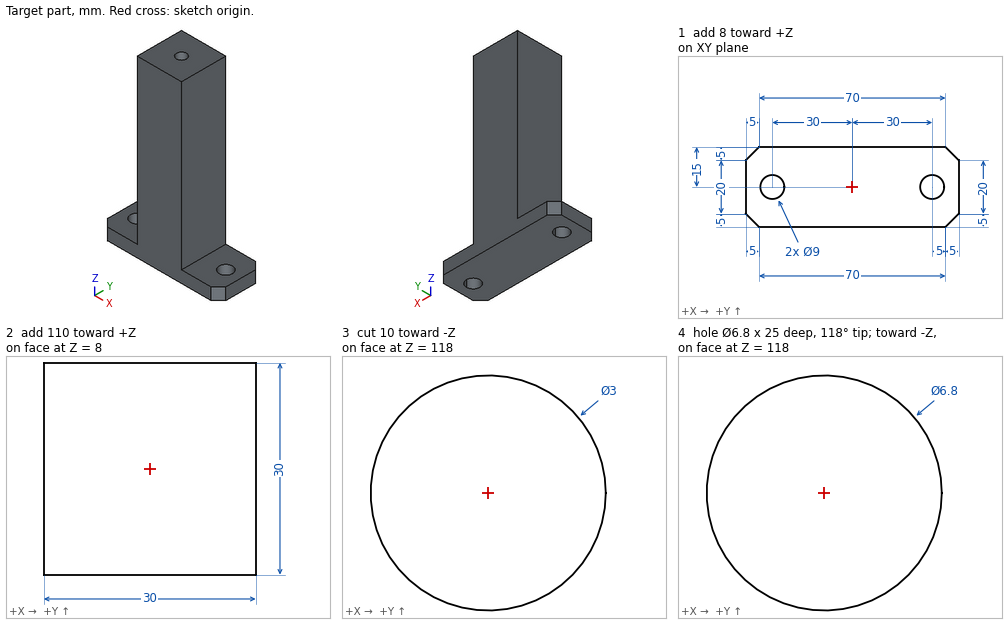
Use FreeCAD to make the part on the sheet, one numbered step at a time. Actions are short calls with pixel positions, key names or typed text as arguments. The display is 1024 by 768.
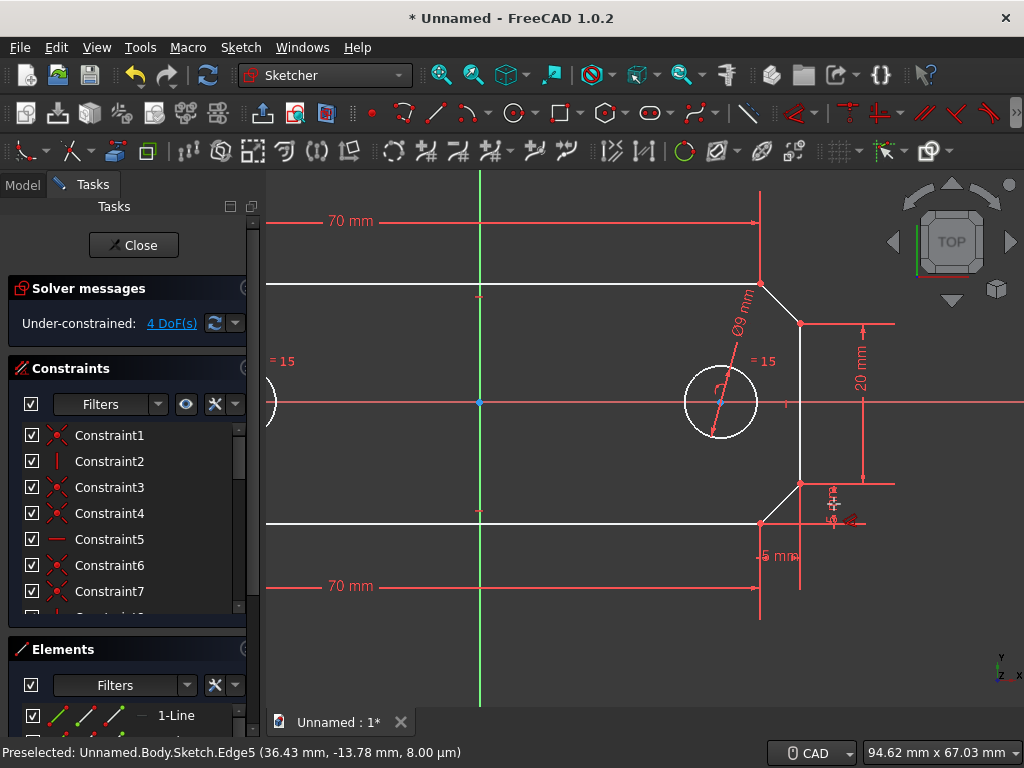
click(721, 402)
click(600, 436)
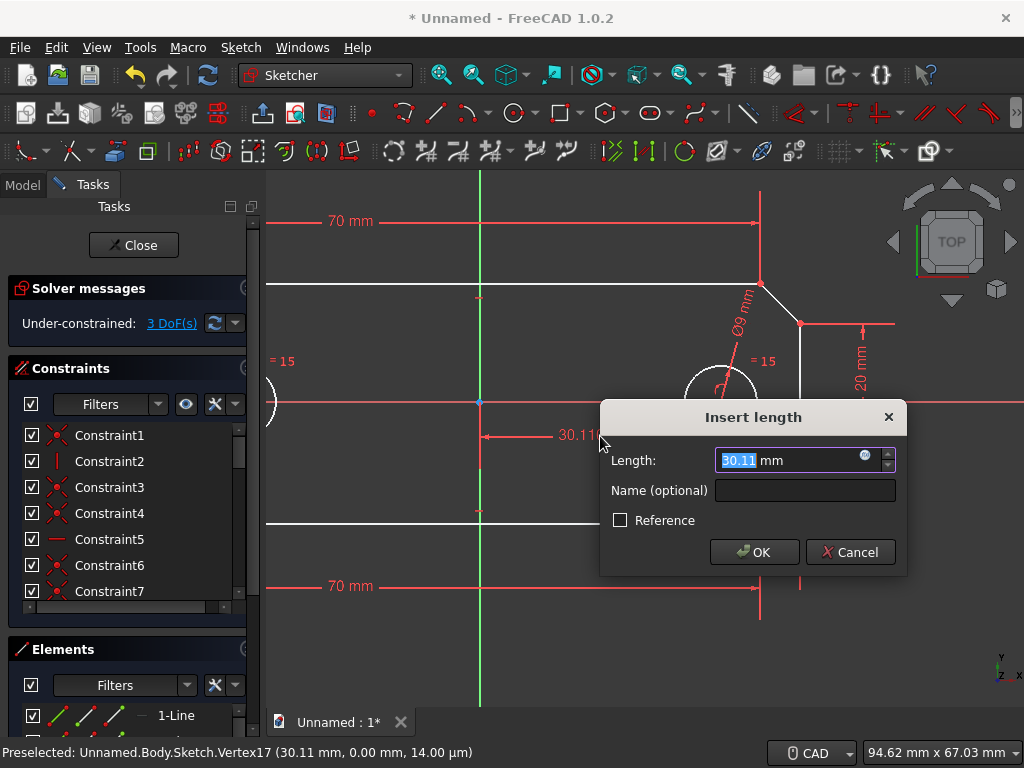
text(30)
key(Return)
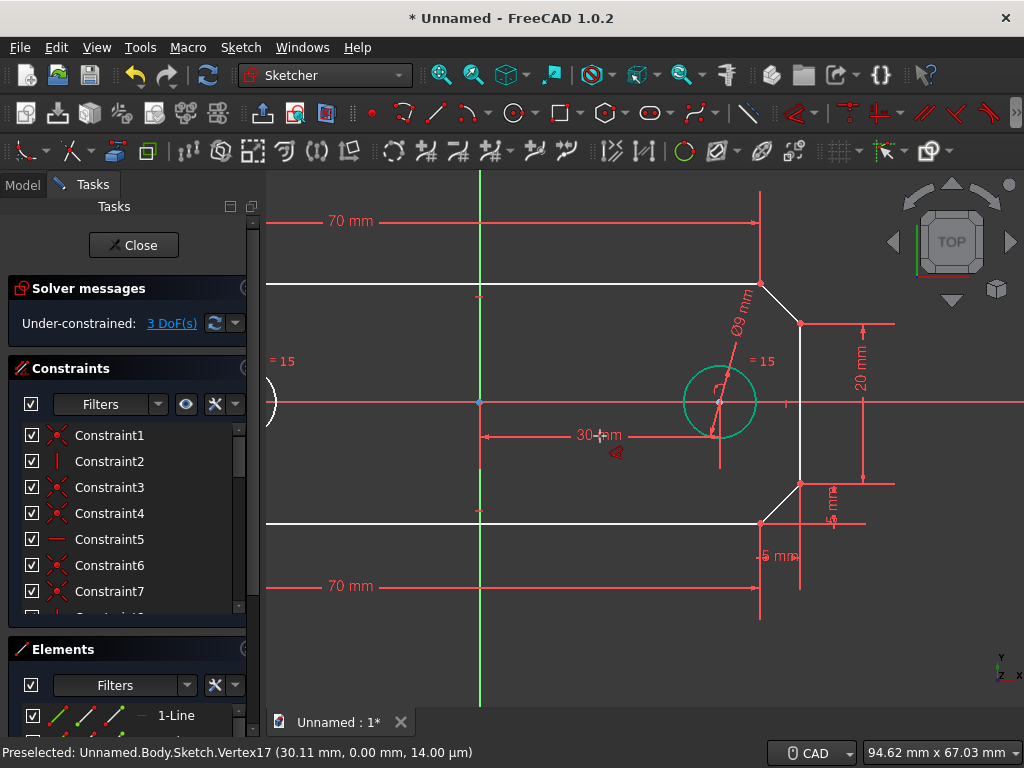
scroll(774, 513, down, 2)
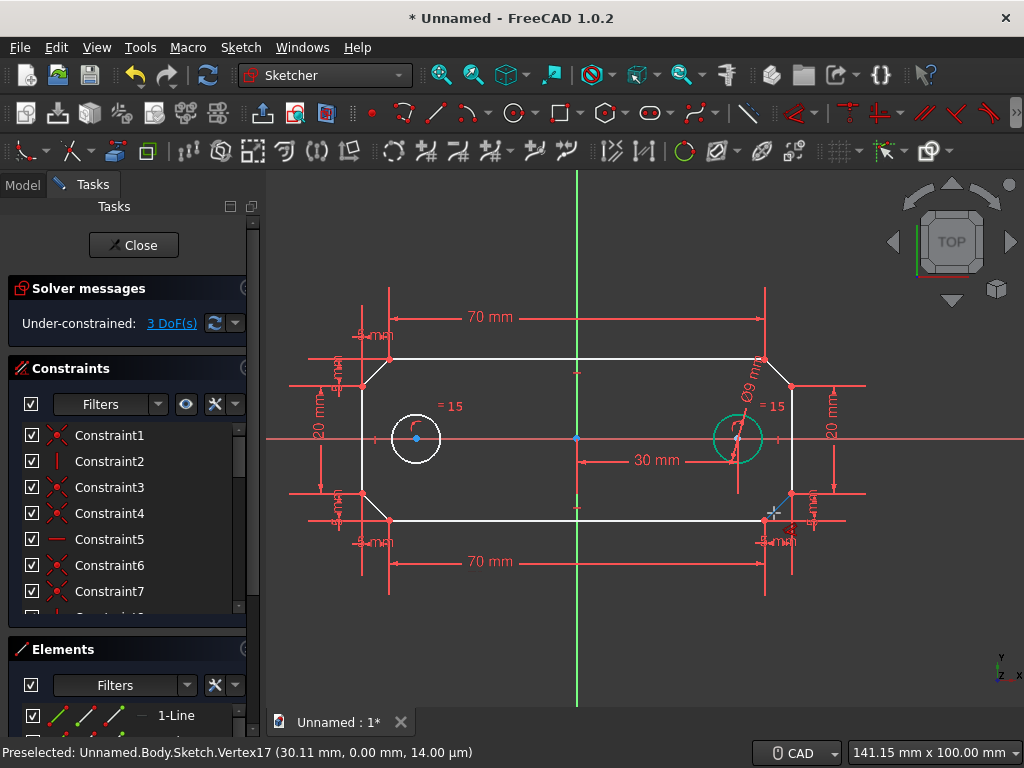
click(416, 439)
click(496, 473)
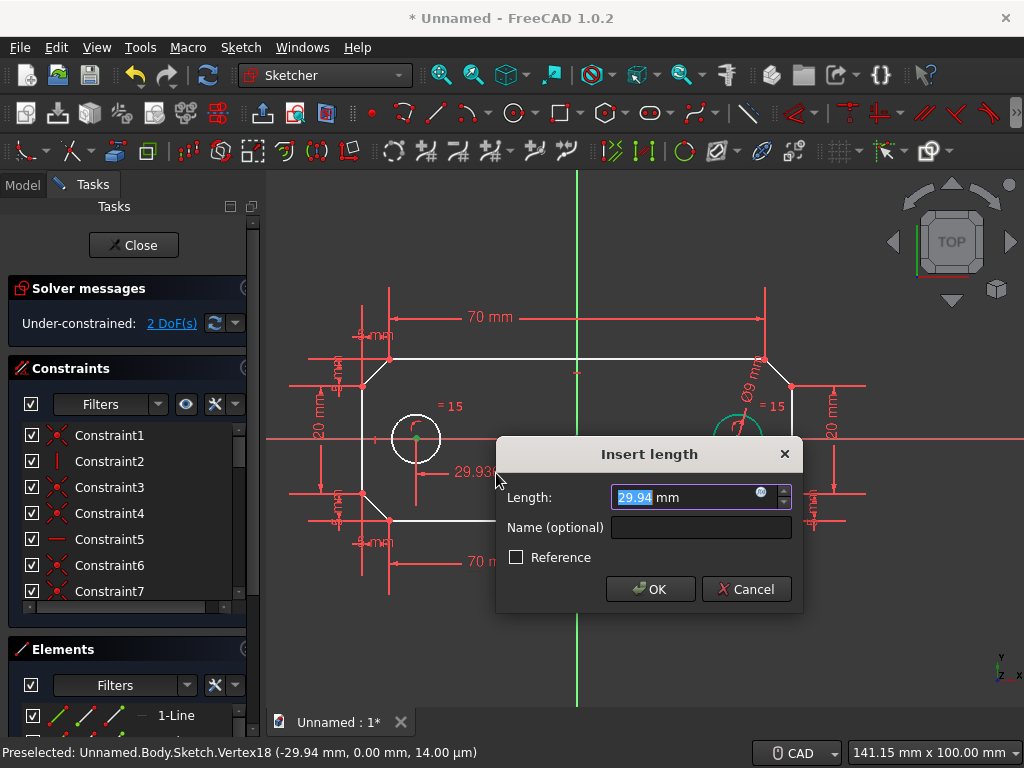
text(30)
key(Return)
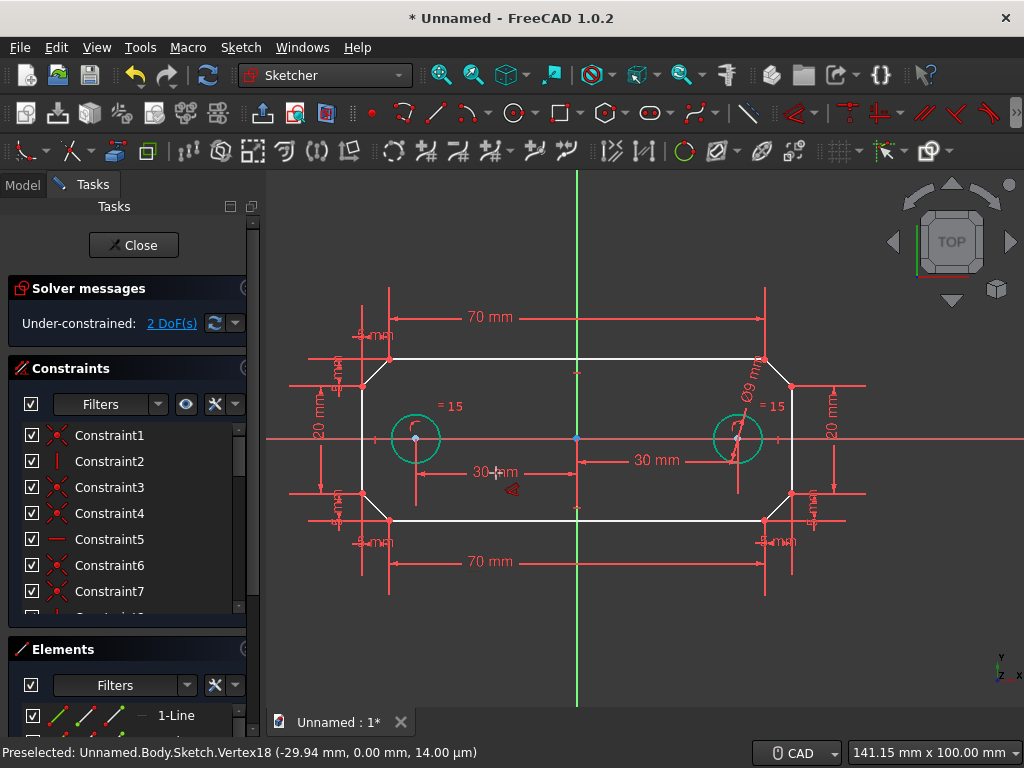
scroll(765, 521, up, 2)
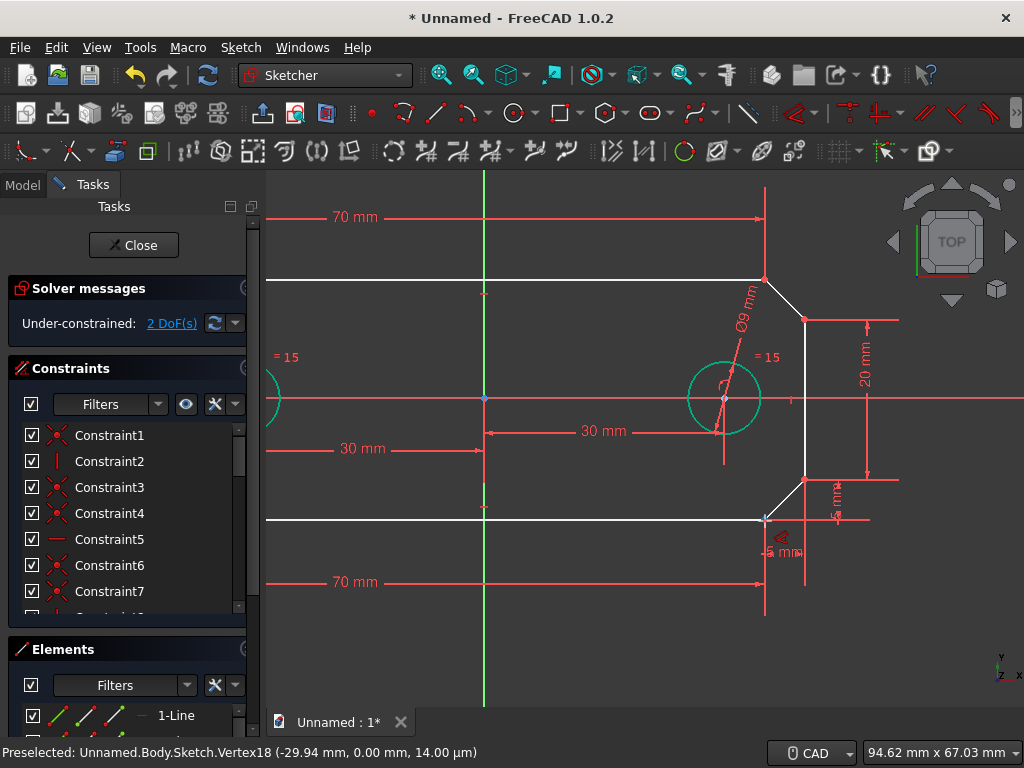
click(765, 520)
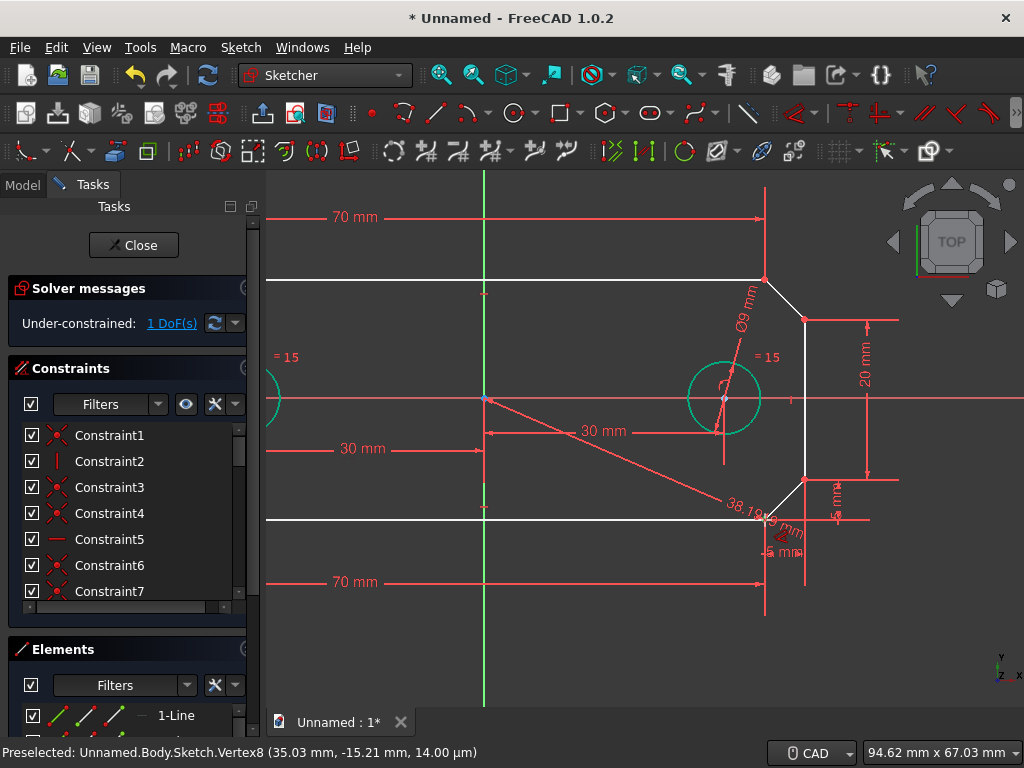
click(724, 398)
click(744, 578)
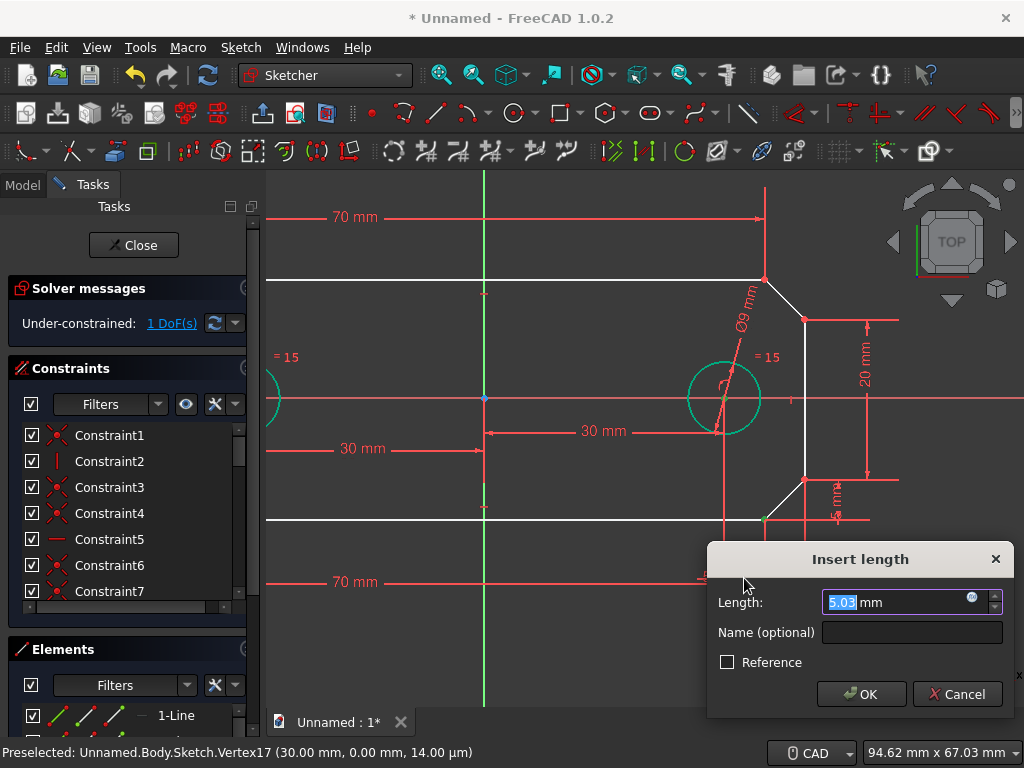
text(5)
key(Return)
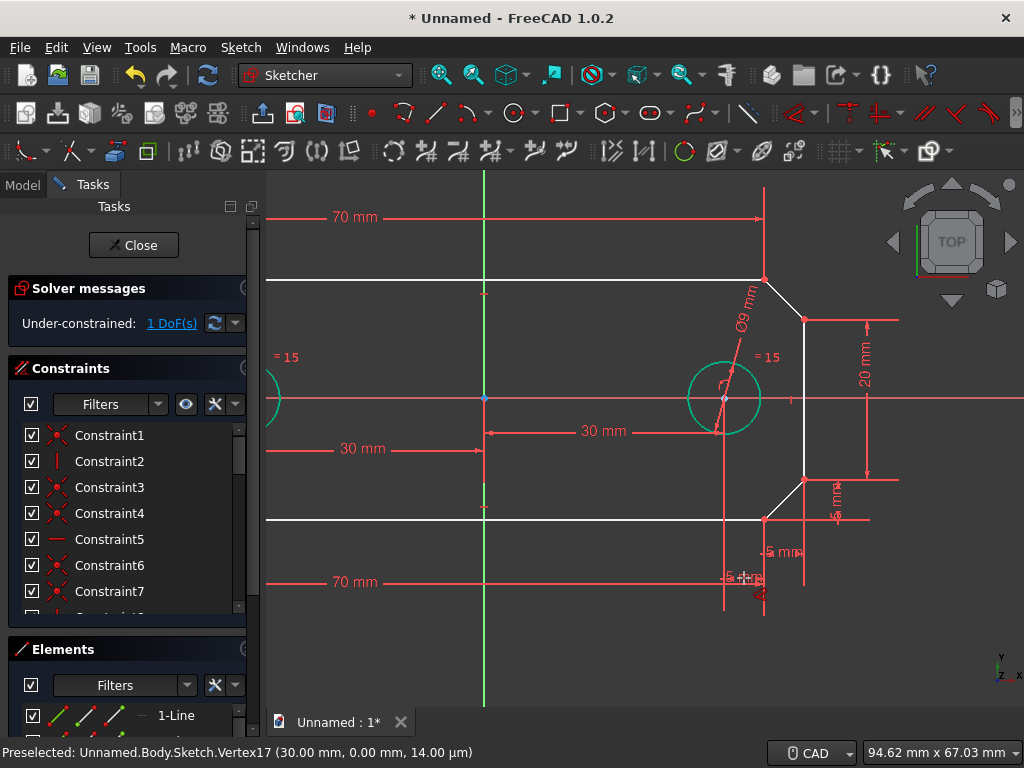
scroll(765, 521, down, 2)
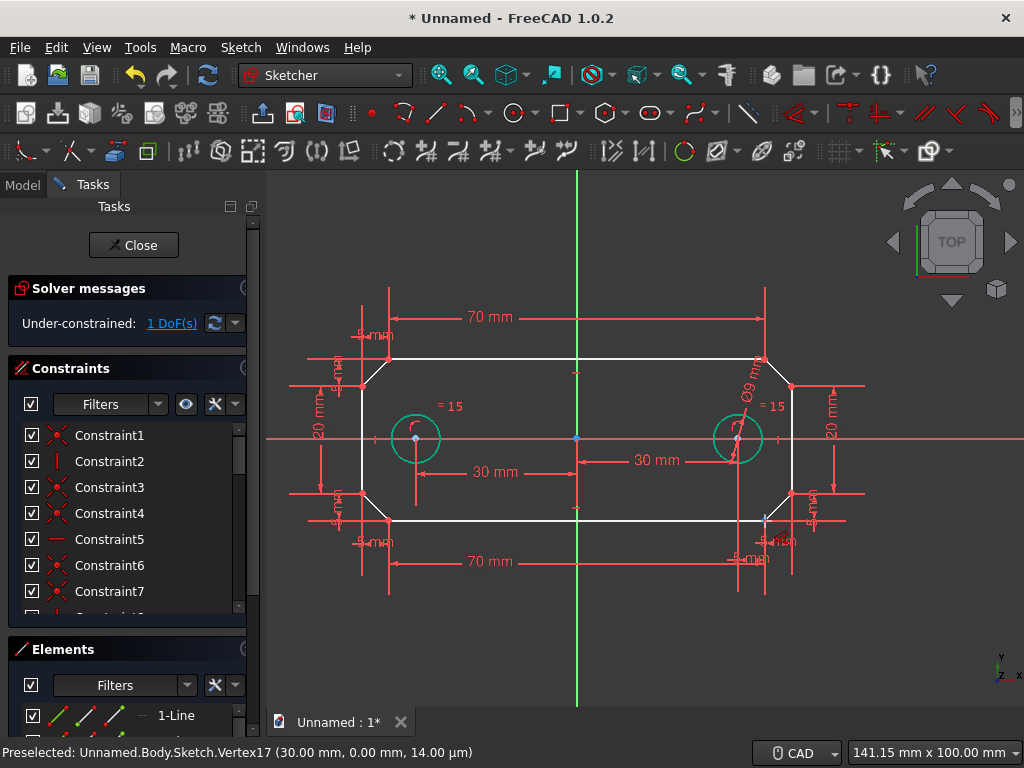
click(389, 359)
click(611, 399)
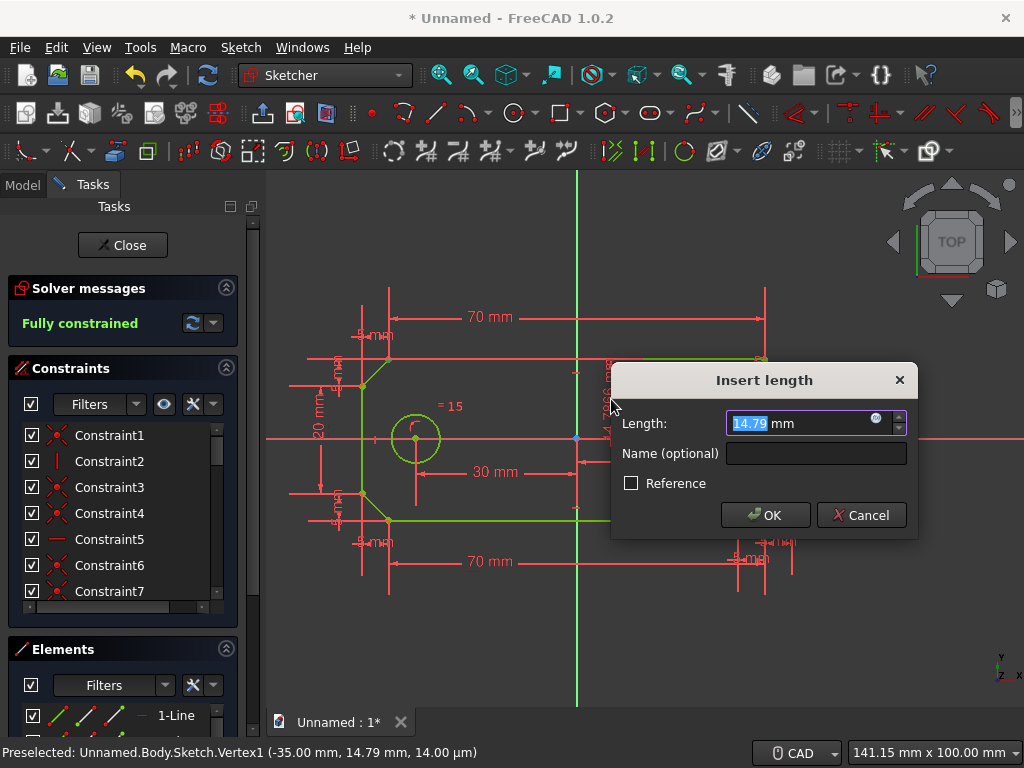
text(15)
key(Return)
key(Escape)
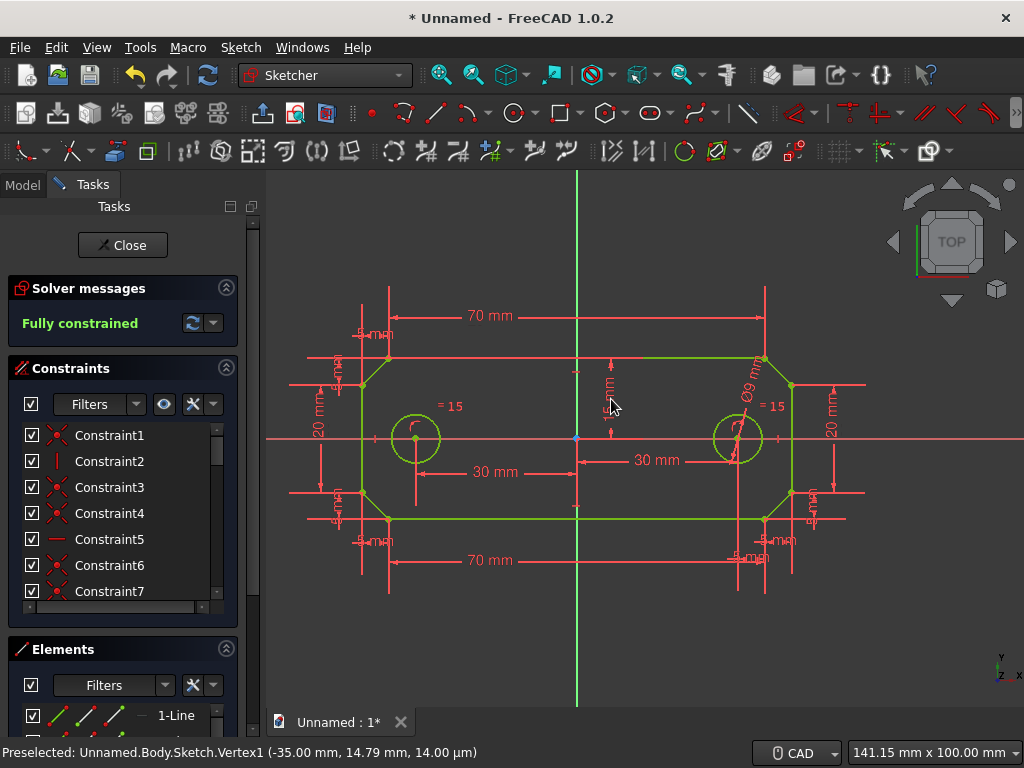
click(123, 245)